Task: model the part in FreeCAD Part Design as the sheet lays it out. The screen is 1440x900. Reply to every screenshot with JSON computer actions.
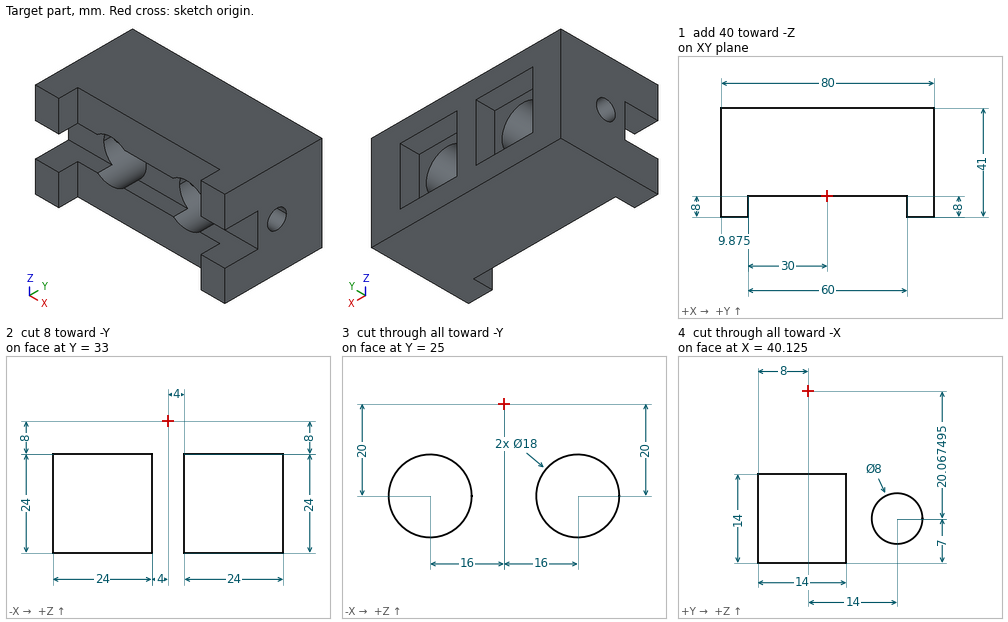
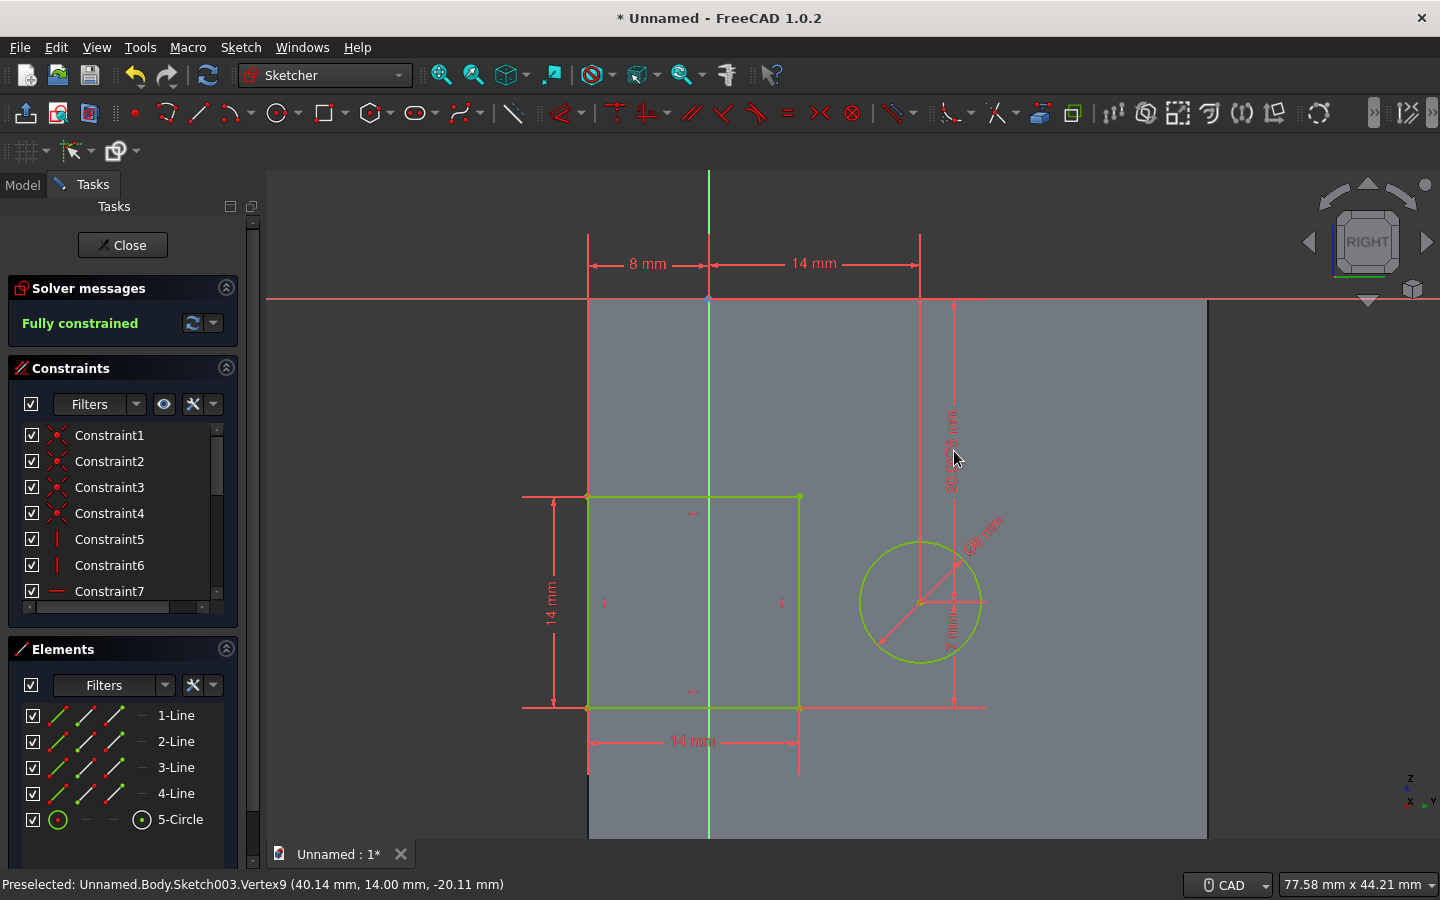
{"action": "left_click", "coordinate": [123, 245]}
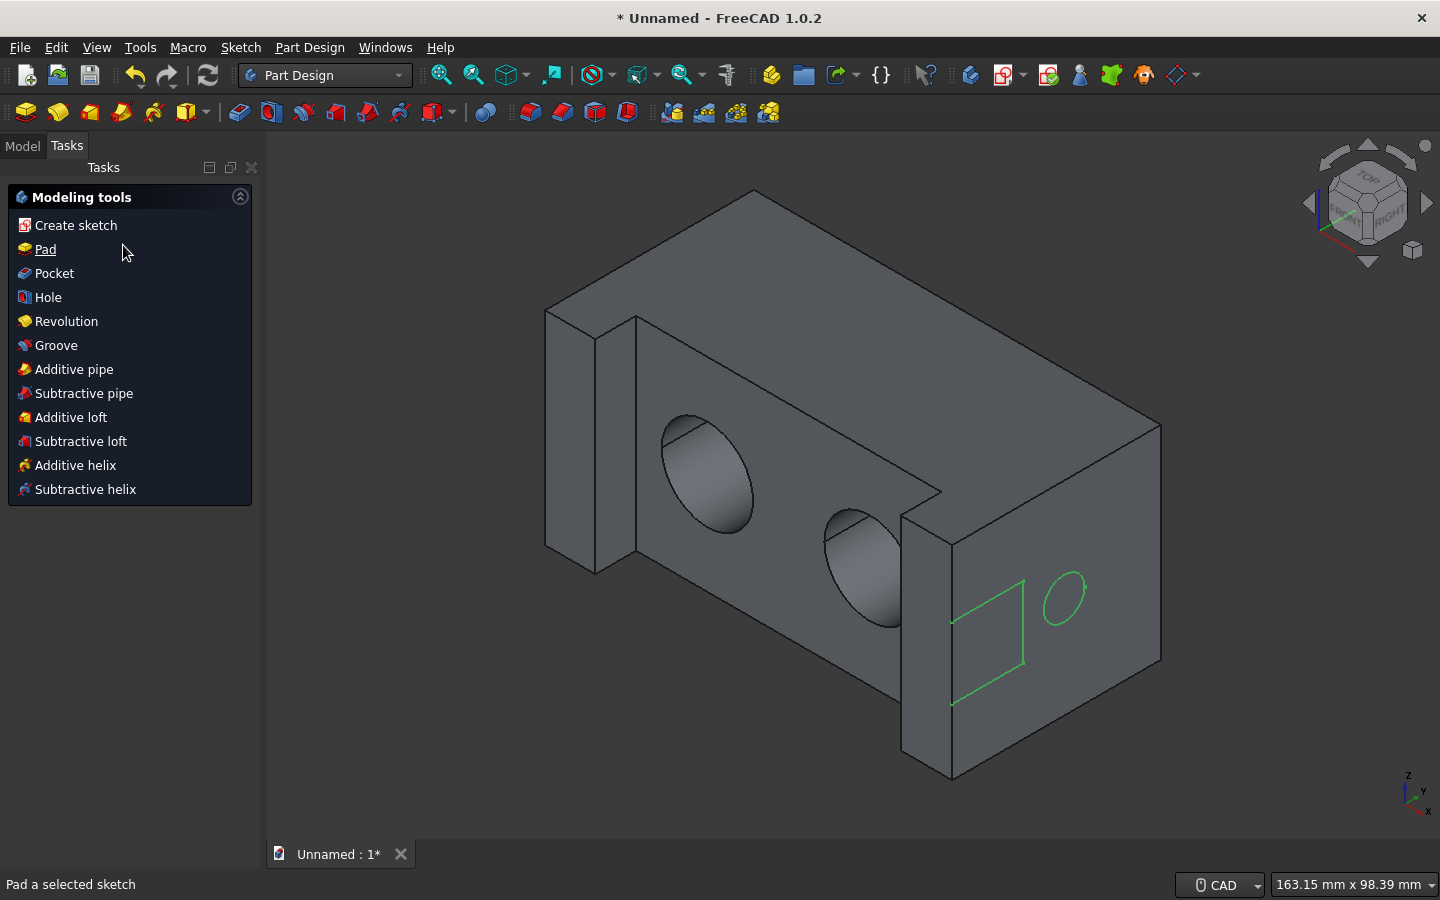
{"action": "left_click", "coordinate": [240, 112]}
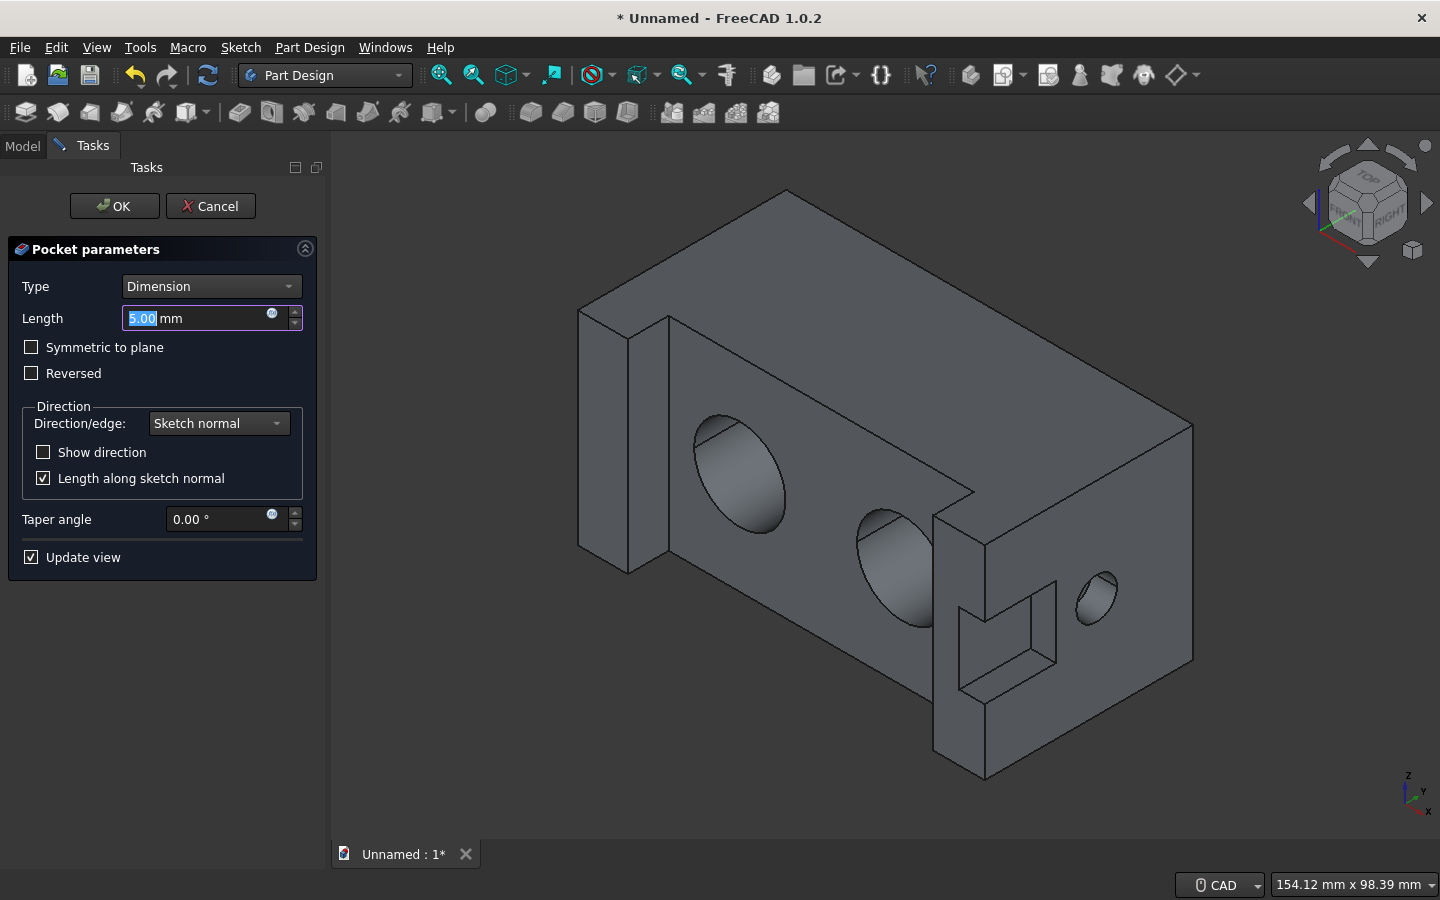
{"action": "left_click", "coordinate": [212, 286]}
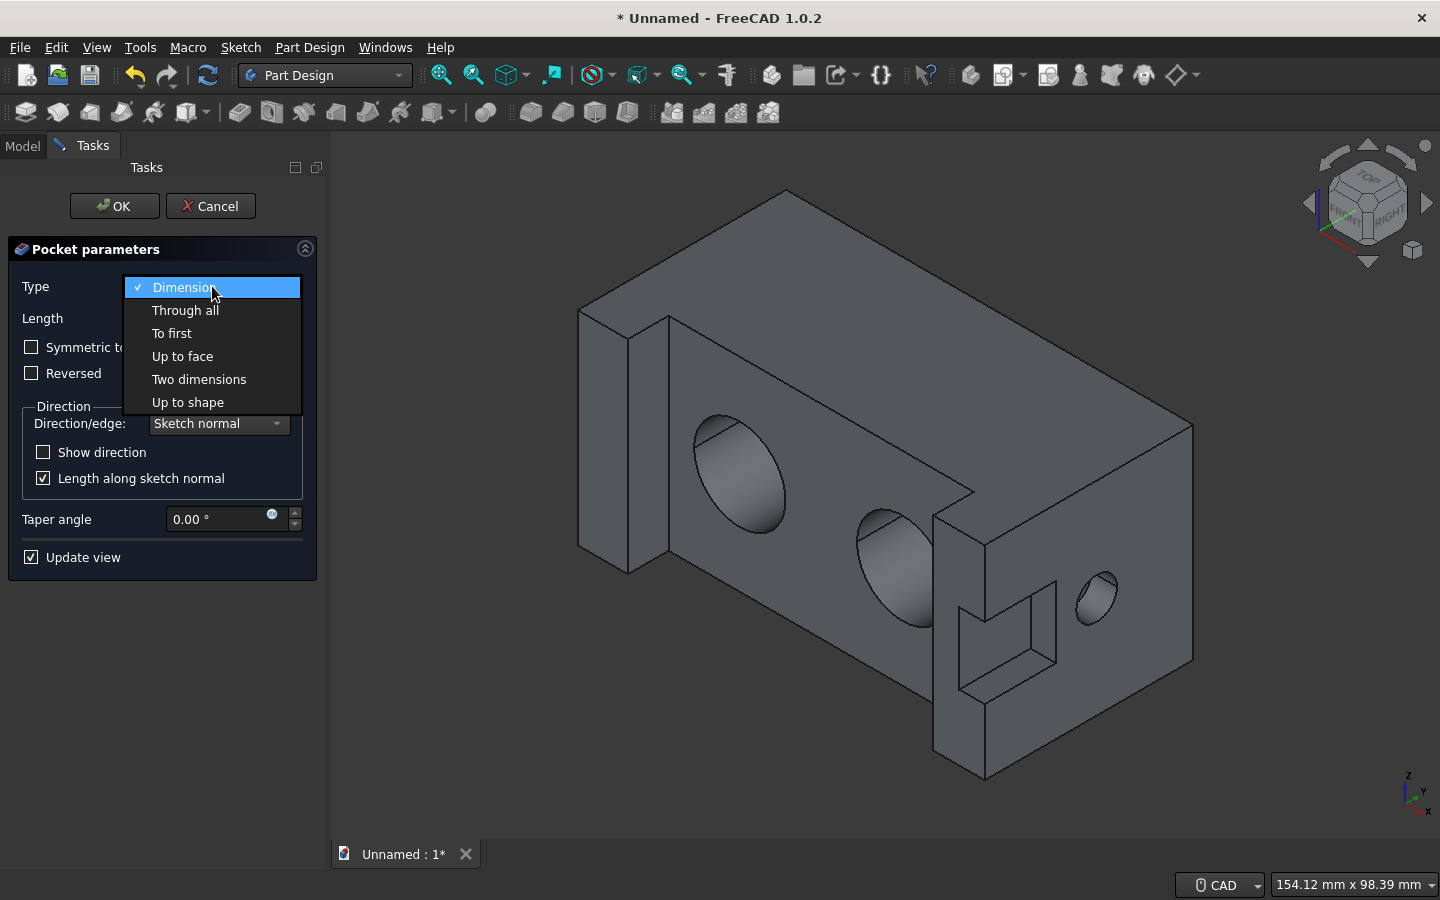
{"action": "left_click", "coordinate": [212, 310]}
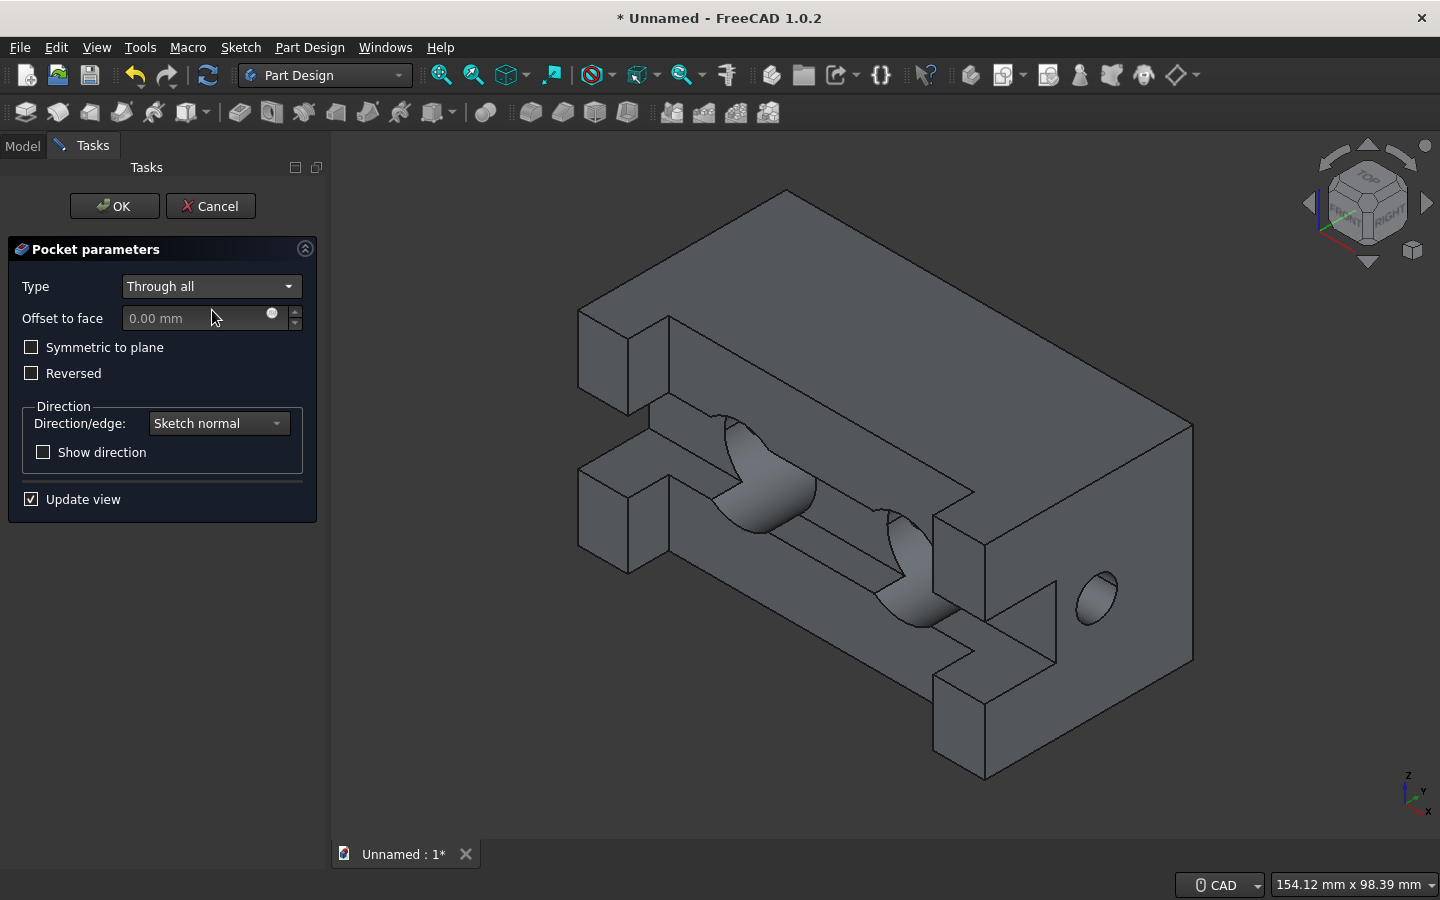
{"action": "left_click", "coordinate": [115, 206]}